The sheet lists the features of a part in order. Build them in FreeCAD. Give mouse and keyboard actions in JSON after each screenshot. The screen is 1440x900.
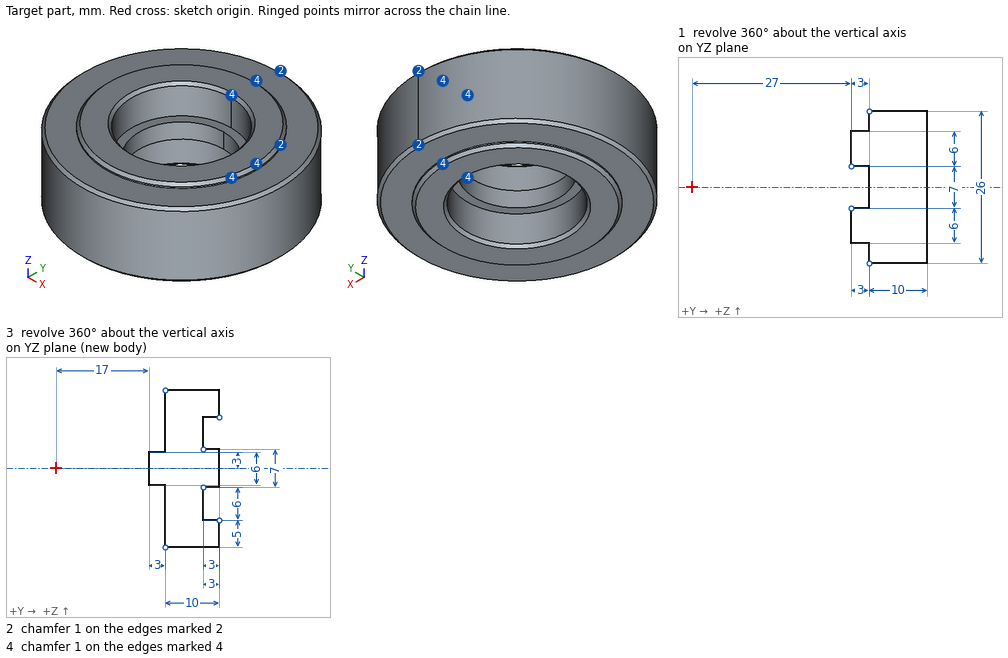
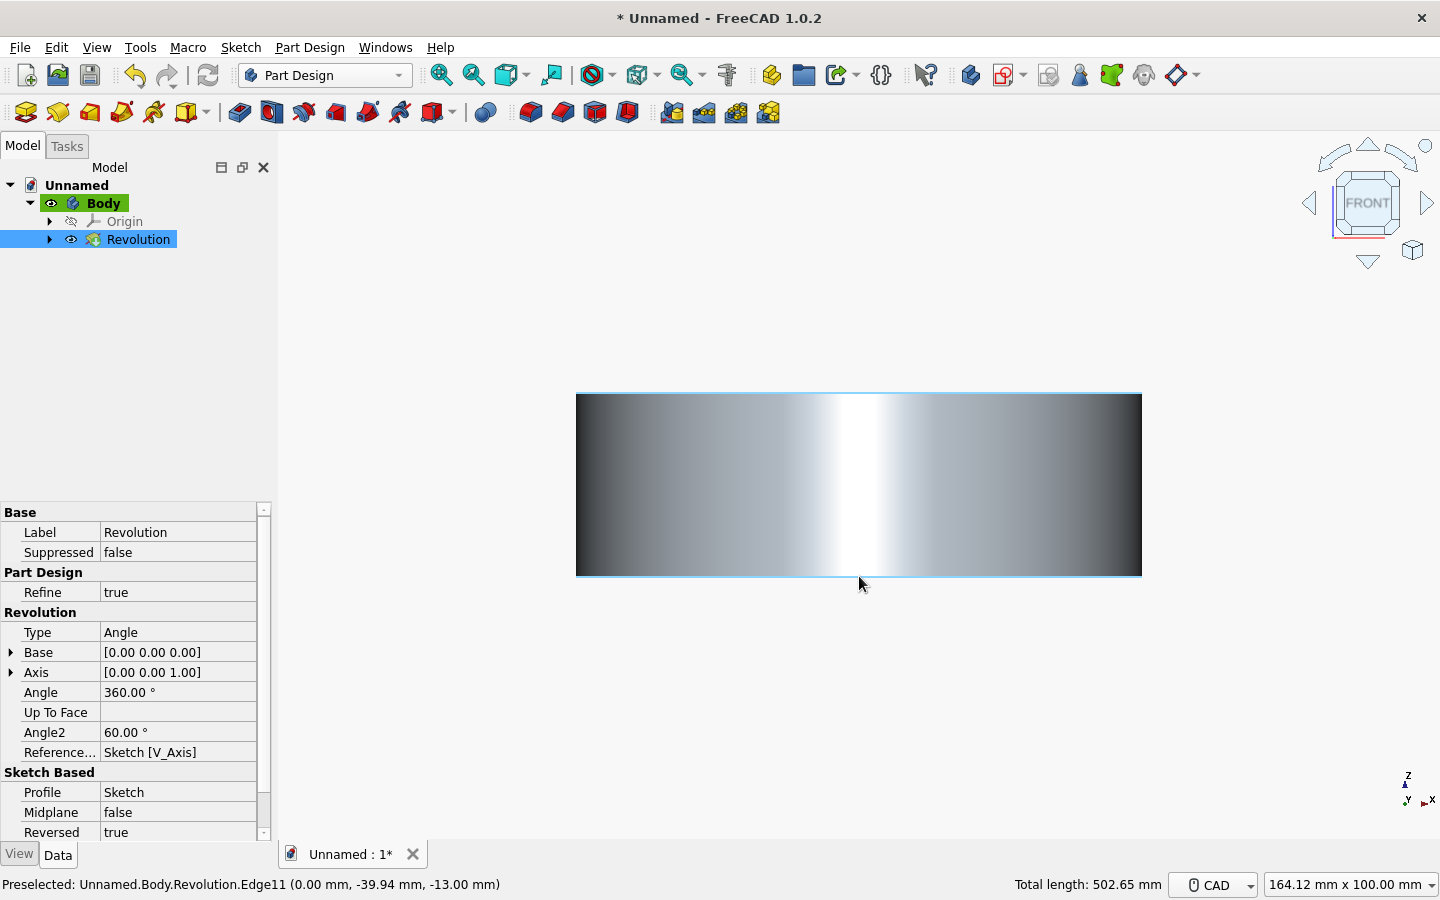
{"action": "left_click", "coordinate": [564, 112]}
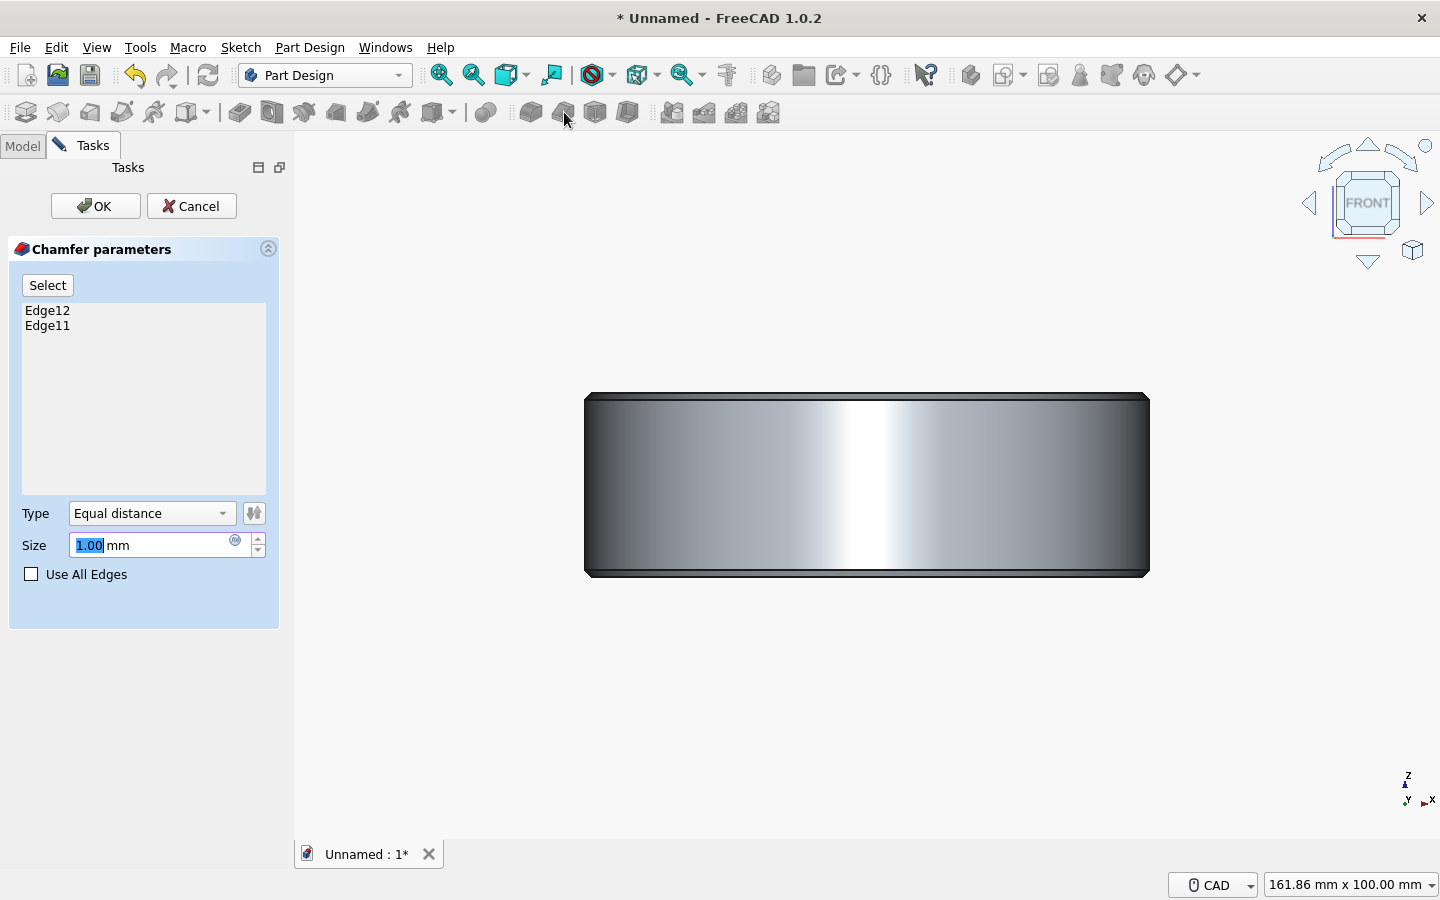
{"action": "type", "text": "1"}
{"action": "key", "text": "Tab"}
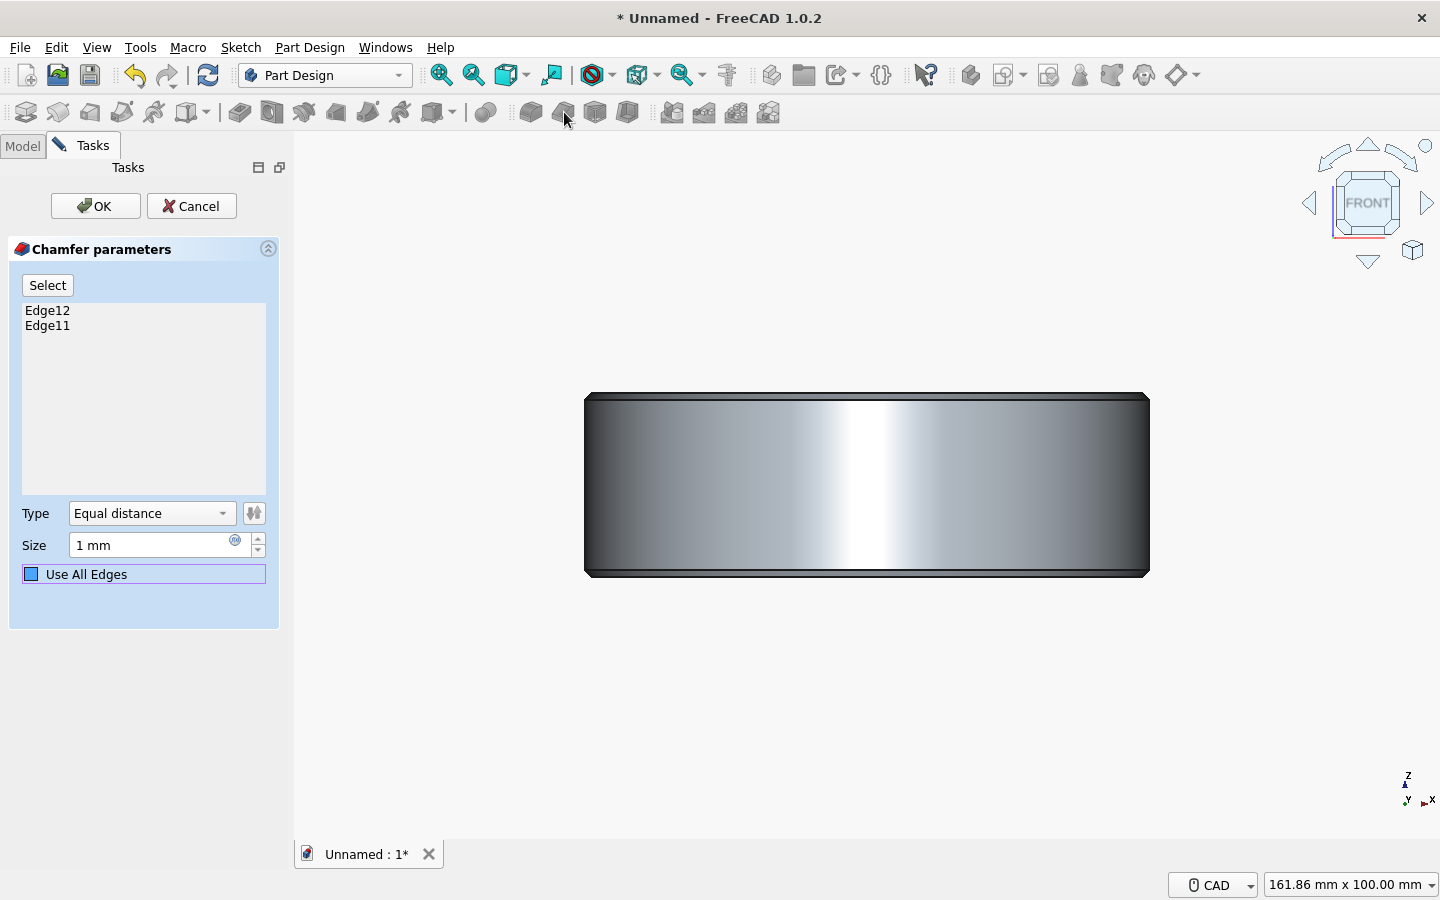
{"action": "left_click", "coordinate": [96, 206]}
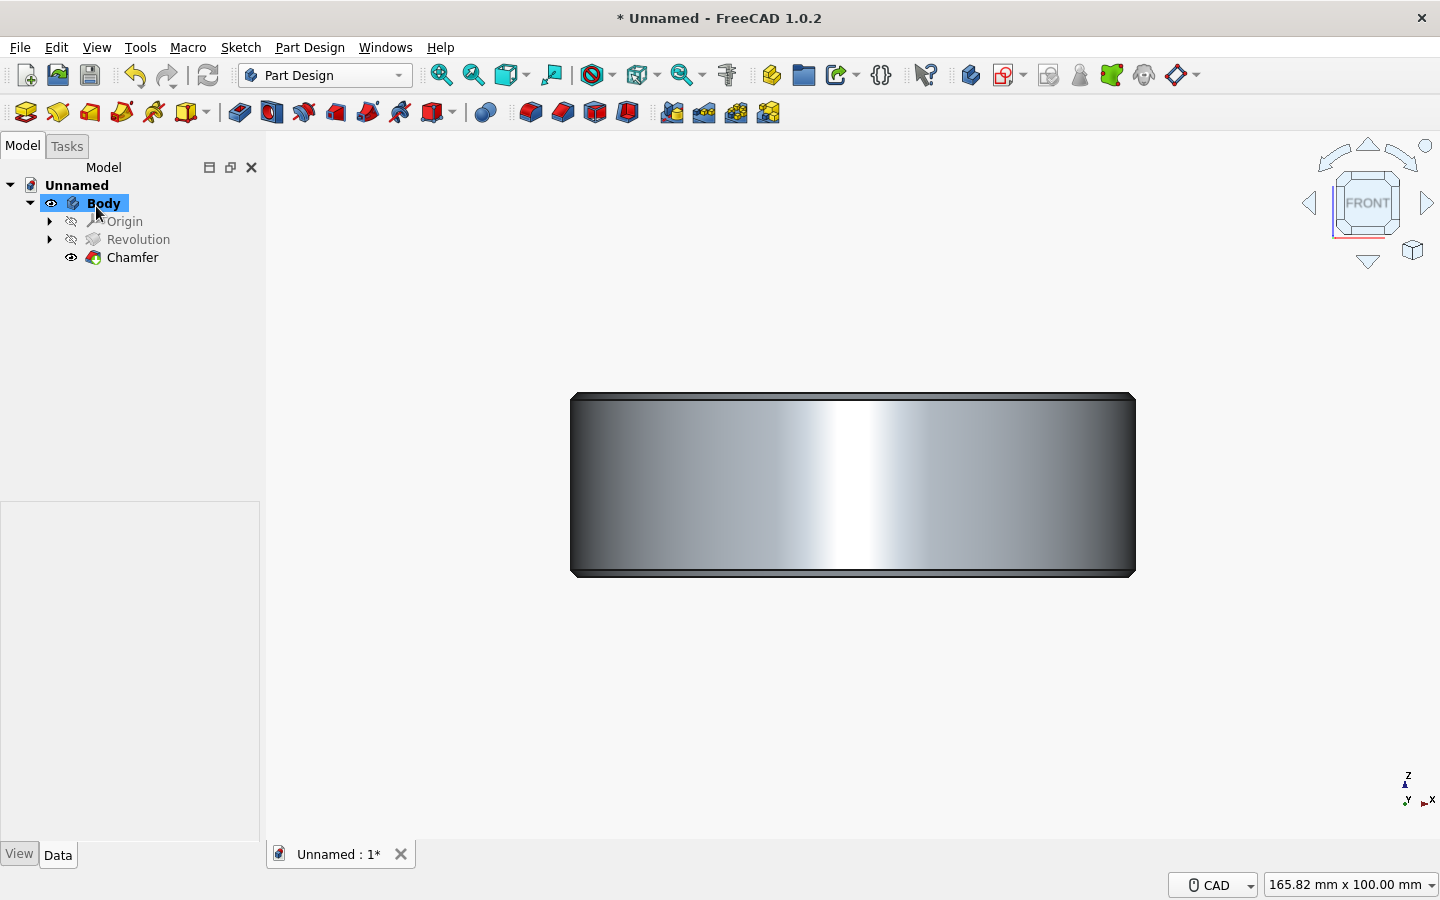
{"action": "left_click", "coordinate": [972, 76]}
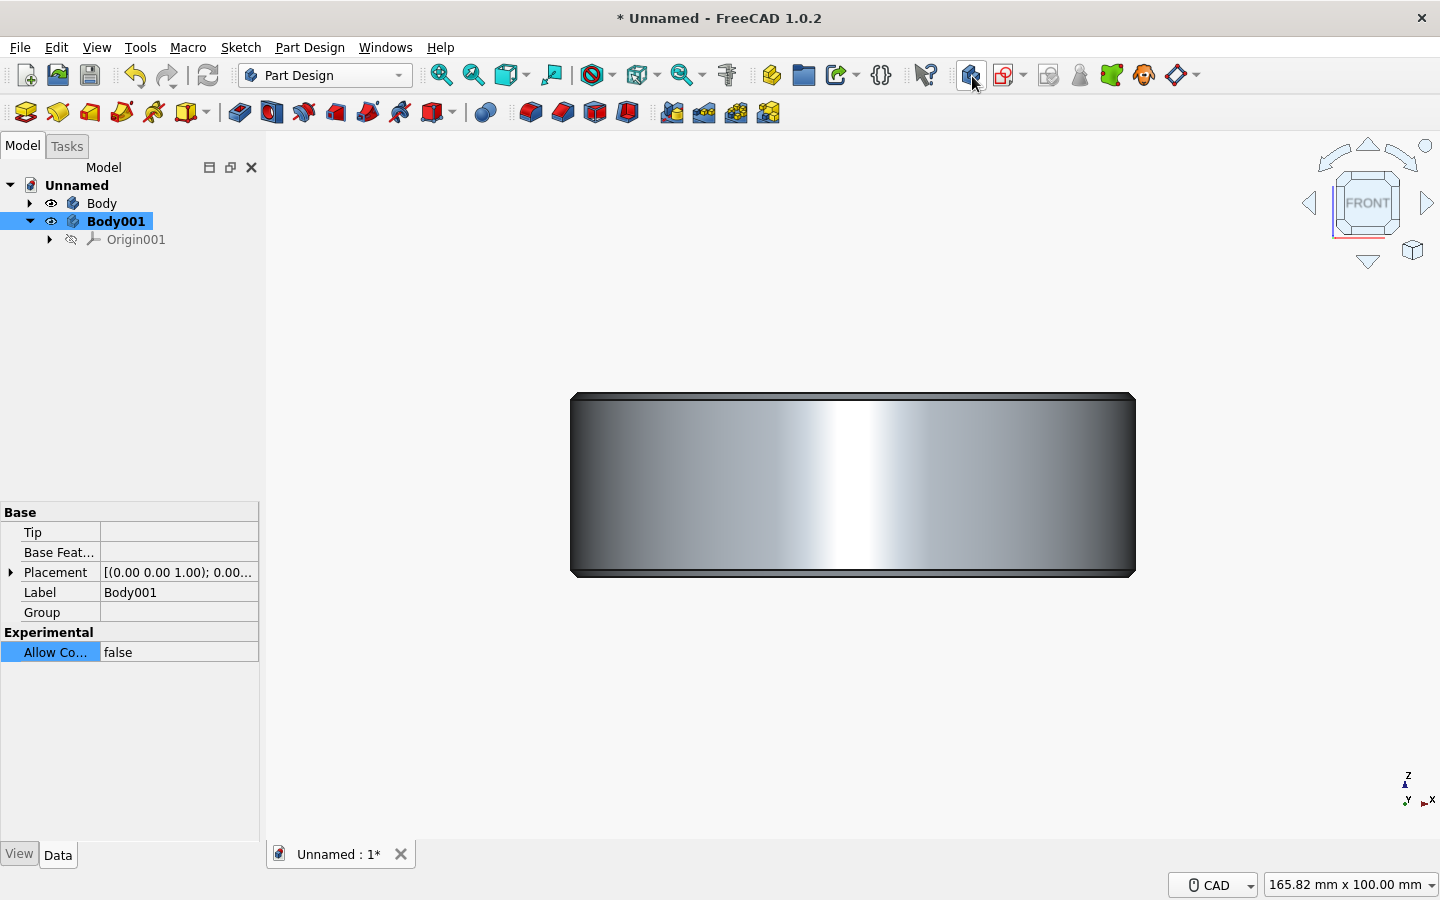
{"action": "left_click", "coordinate": [306, 799]}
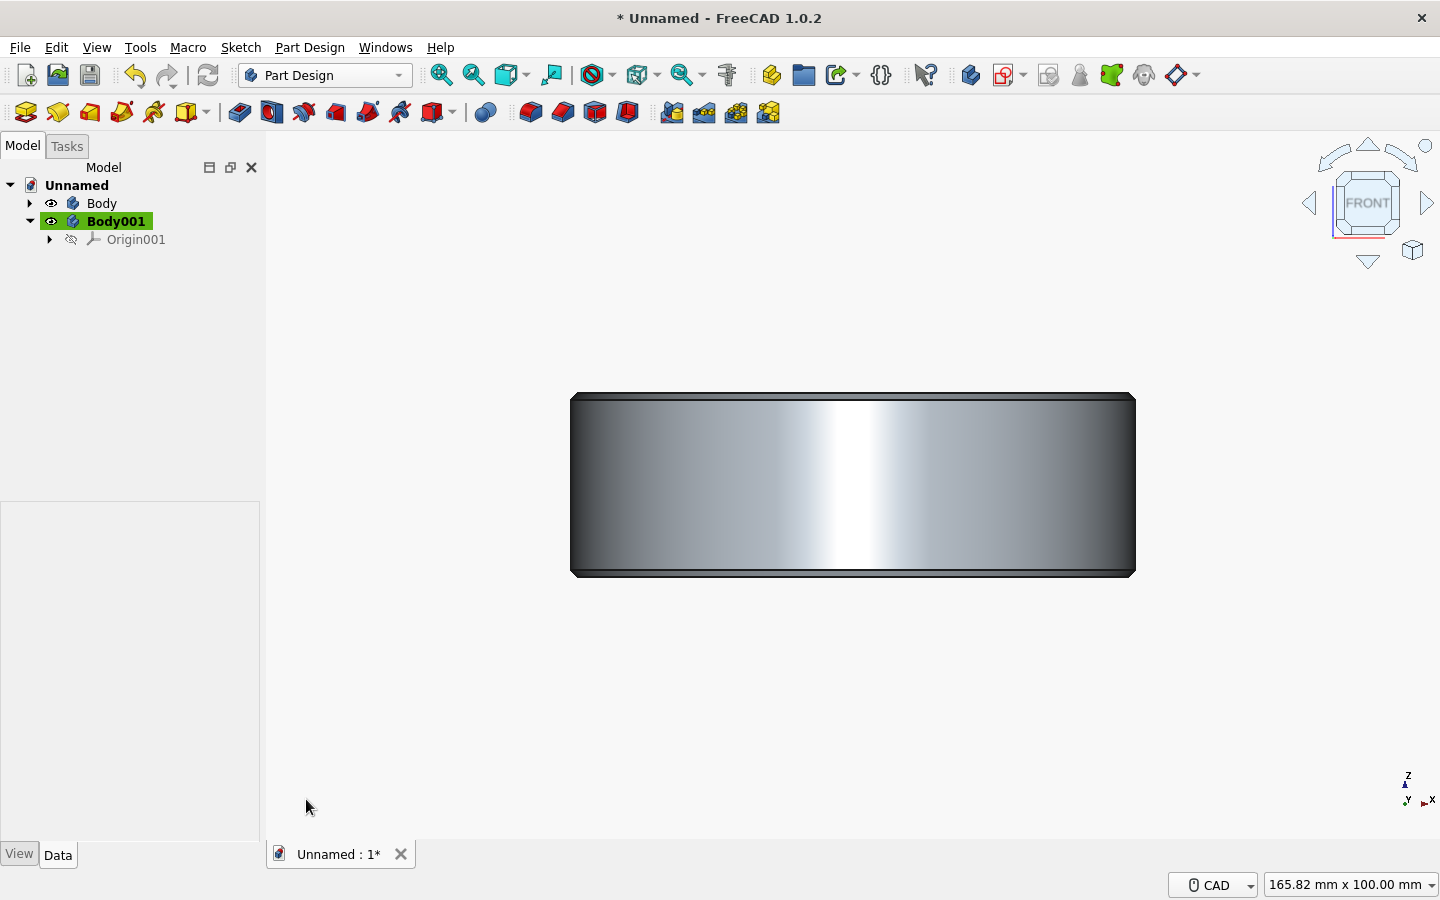
{"action": "left_click", "coordinate": [1004, 76]}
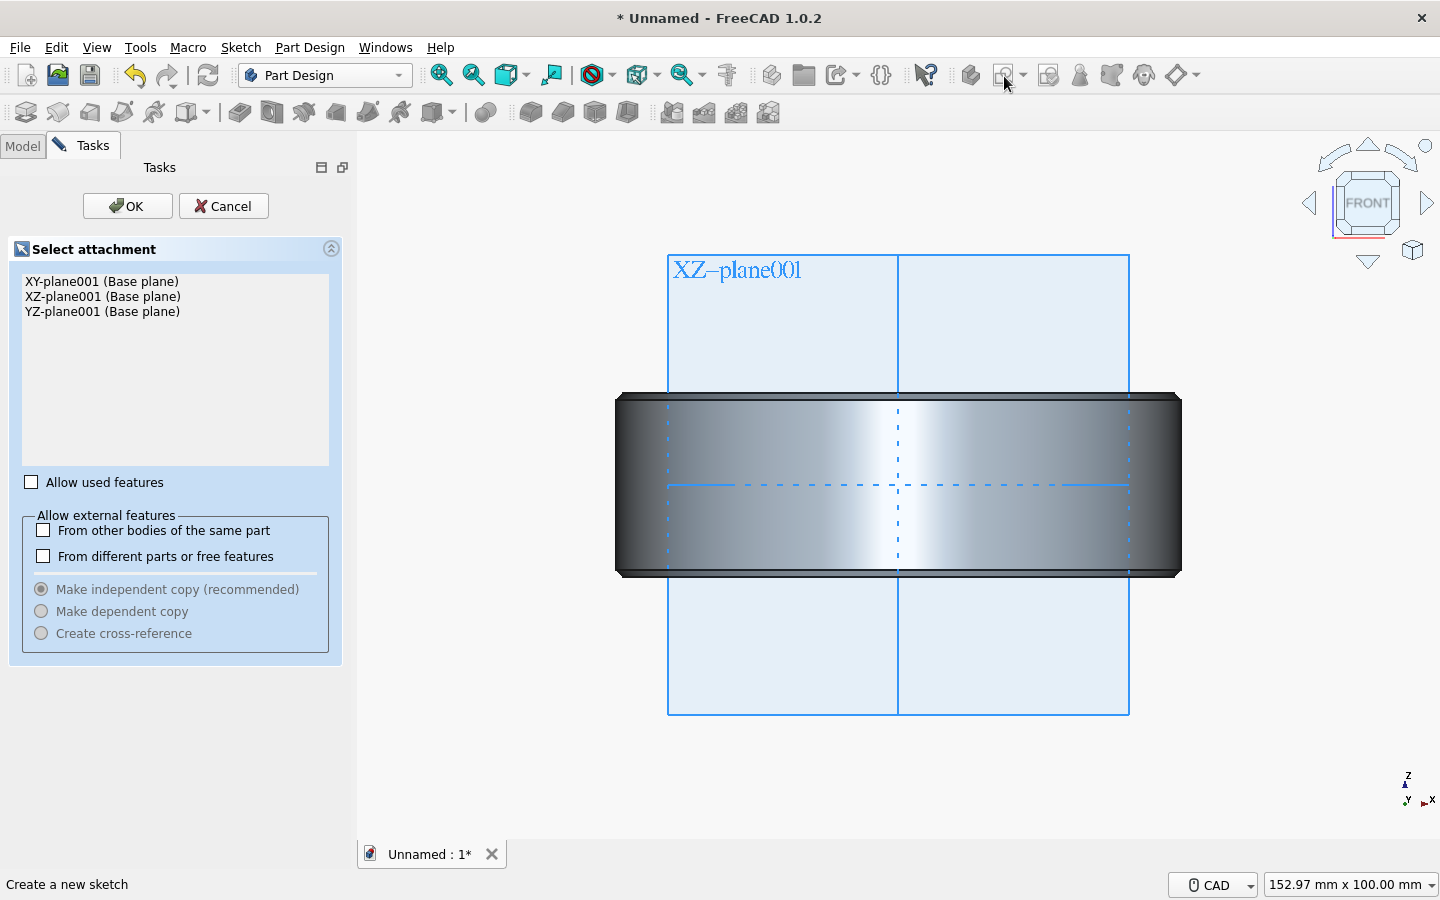
{"action": "left_click", "coordinate": [82, 312]}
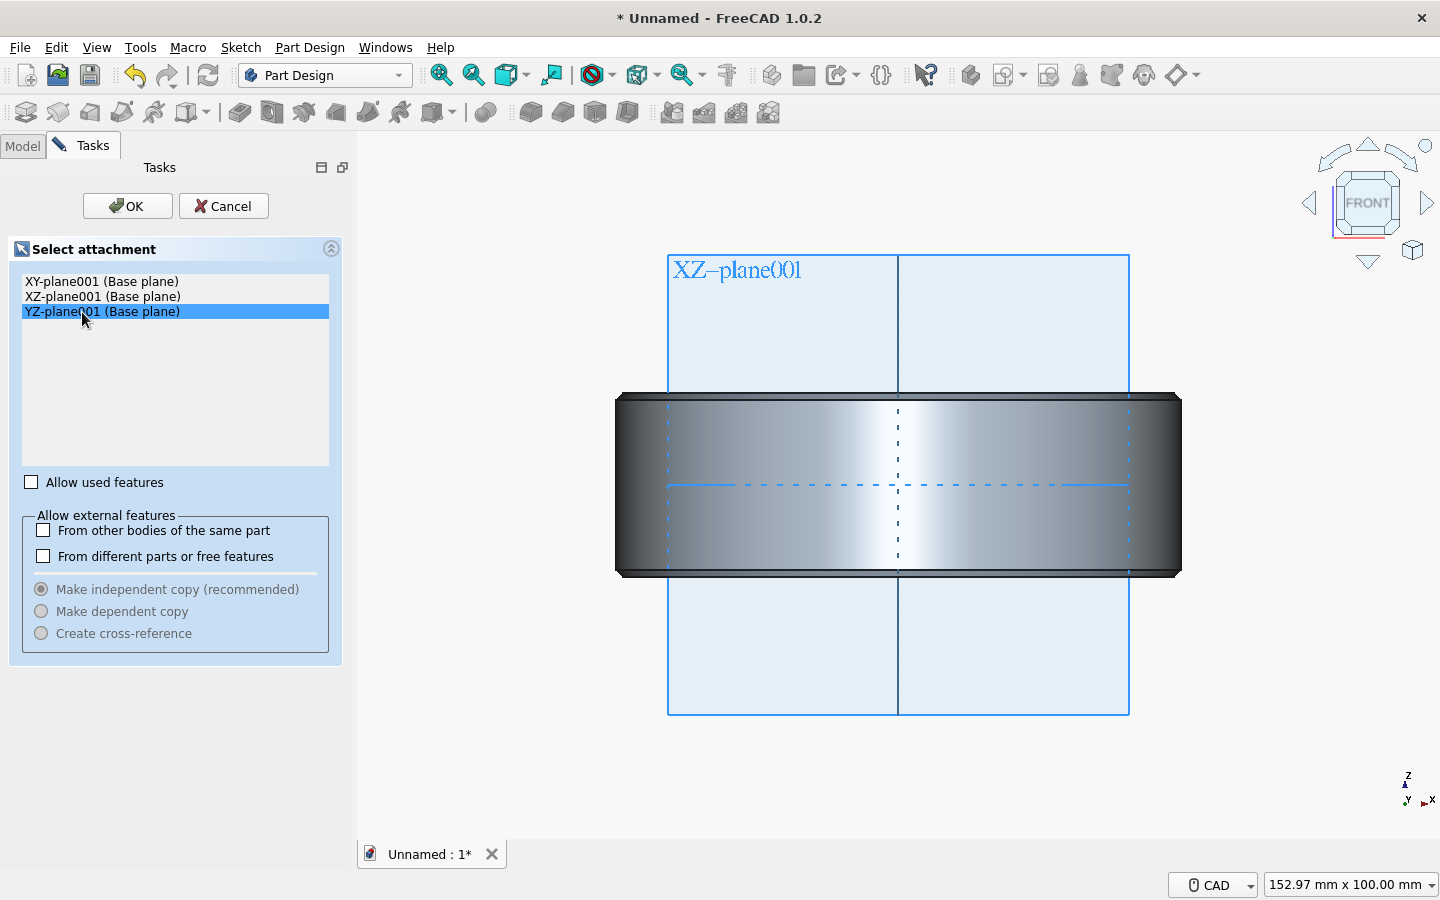
{"action": "left_click", "coordinate": [128, 206]}